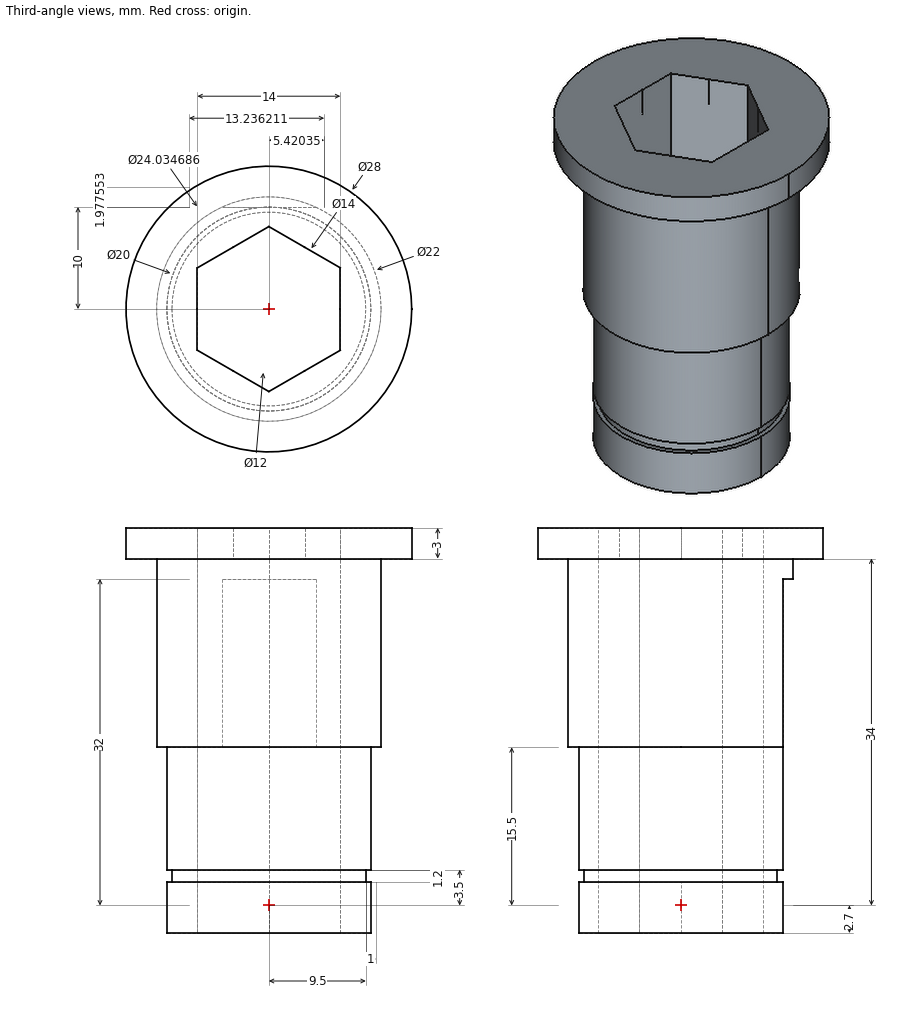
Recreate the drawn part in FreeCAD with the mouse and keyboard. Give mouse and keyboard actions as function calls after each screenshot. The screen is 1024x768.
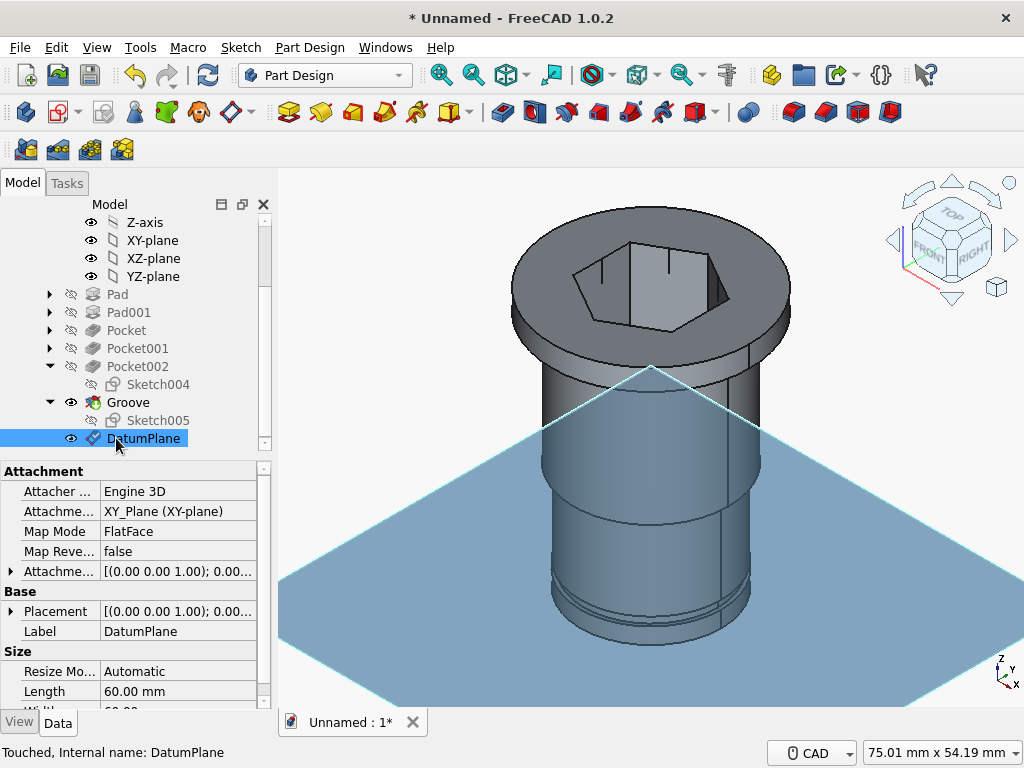
click(58, 112)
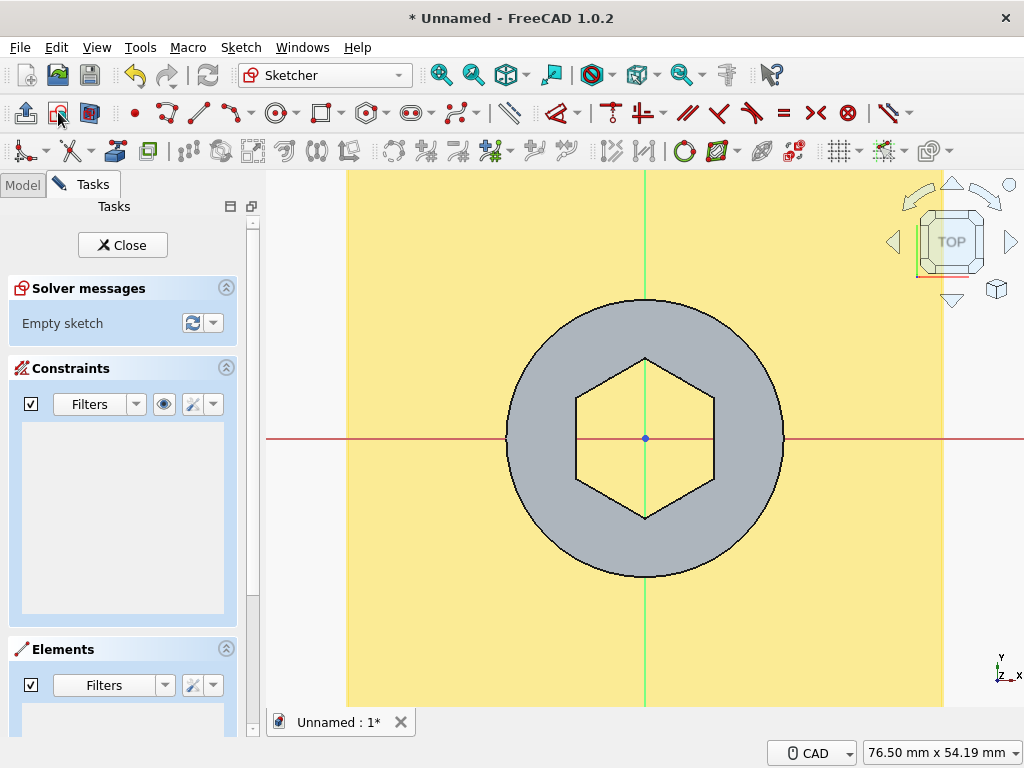
click(90, 114)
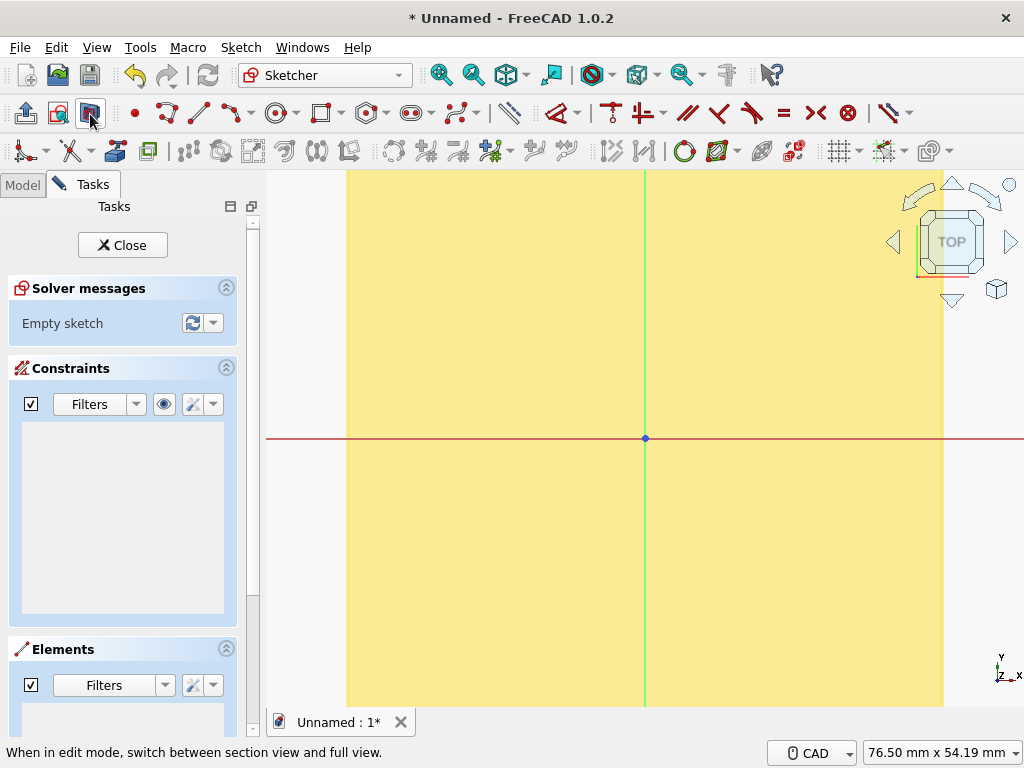
scroll(728, 438, up, 3)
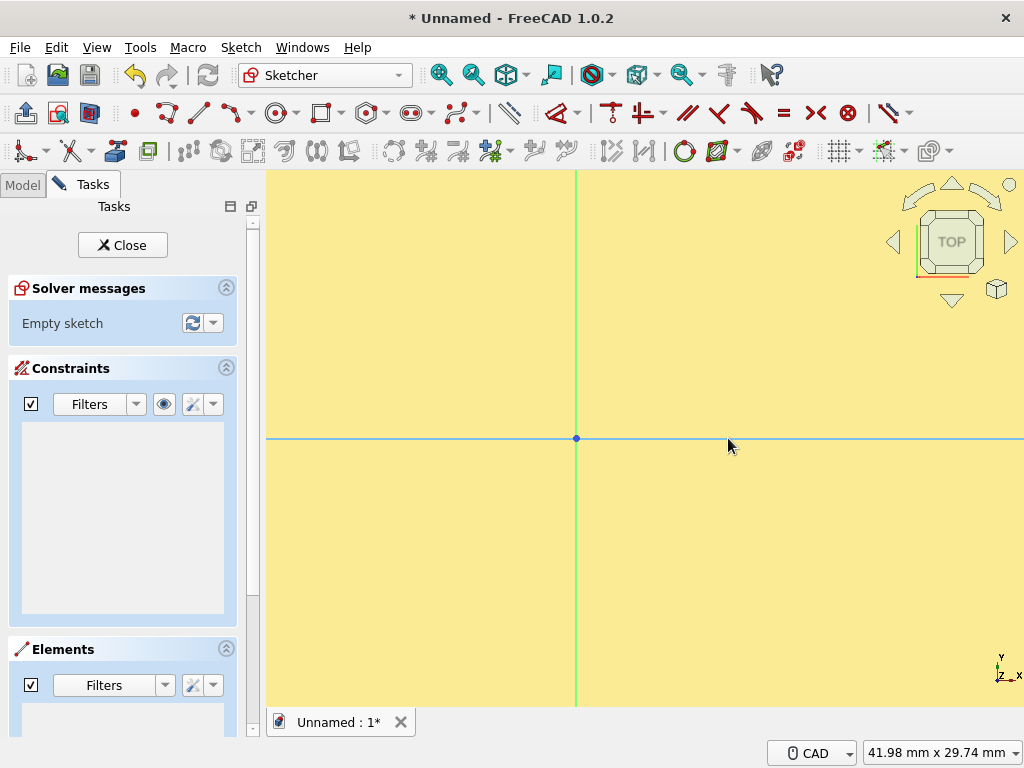
click(366, 114)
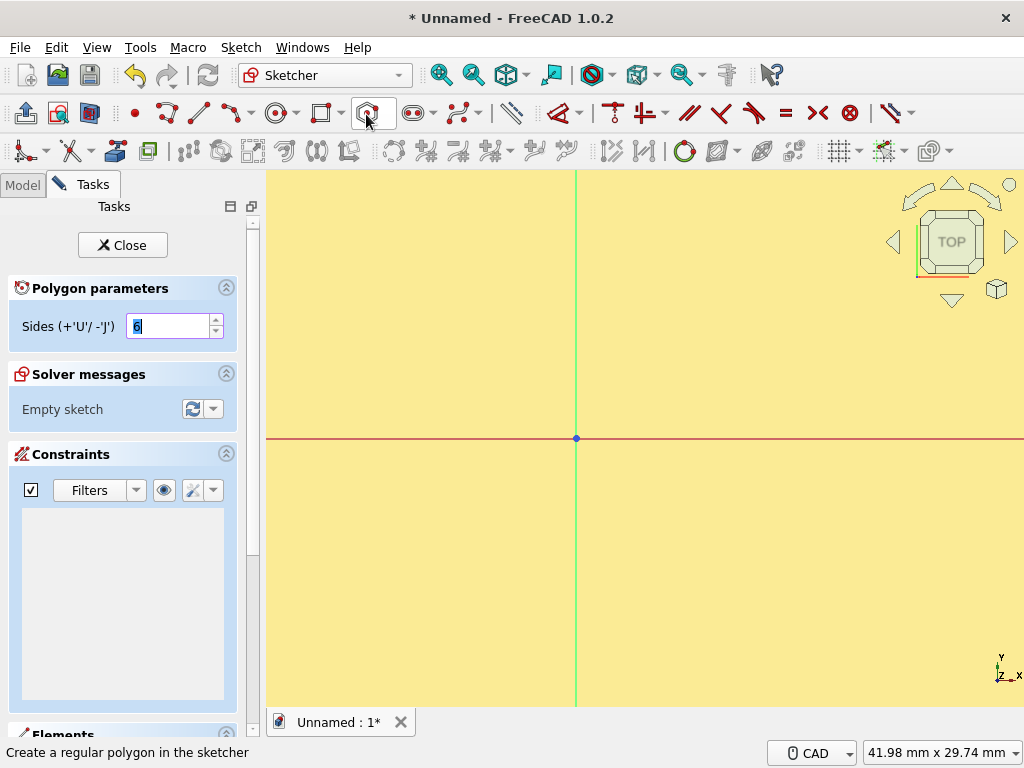
click(576, 438)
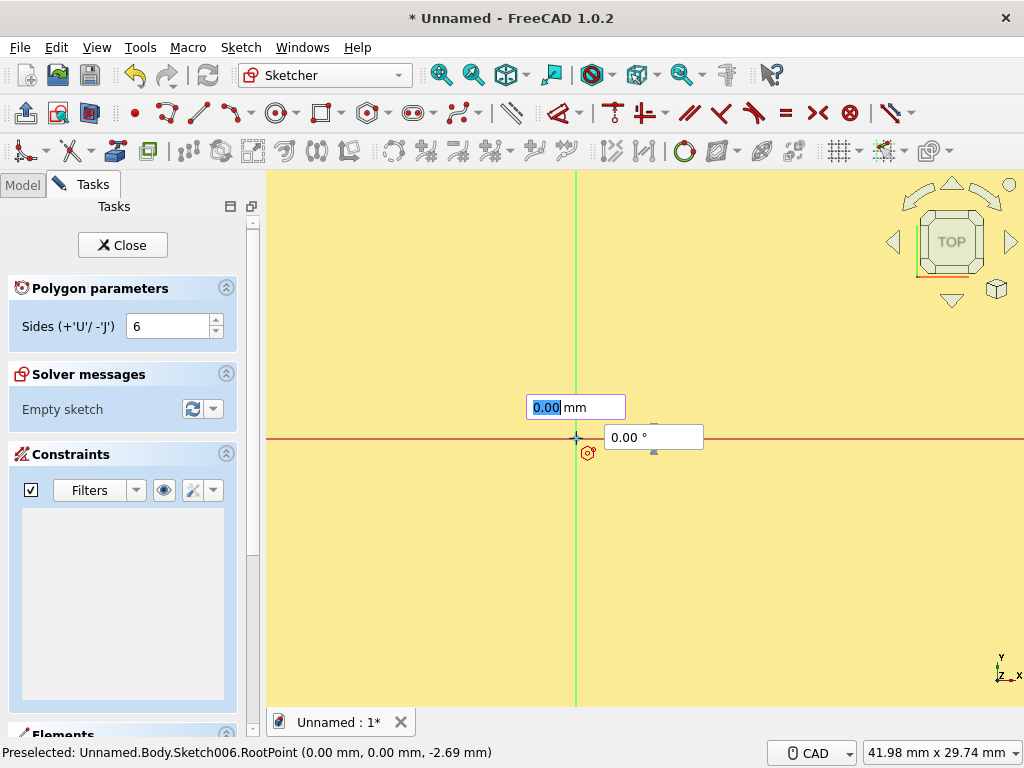
click(576, 584)
right_click(576, 584)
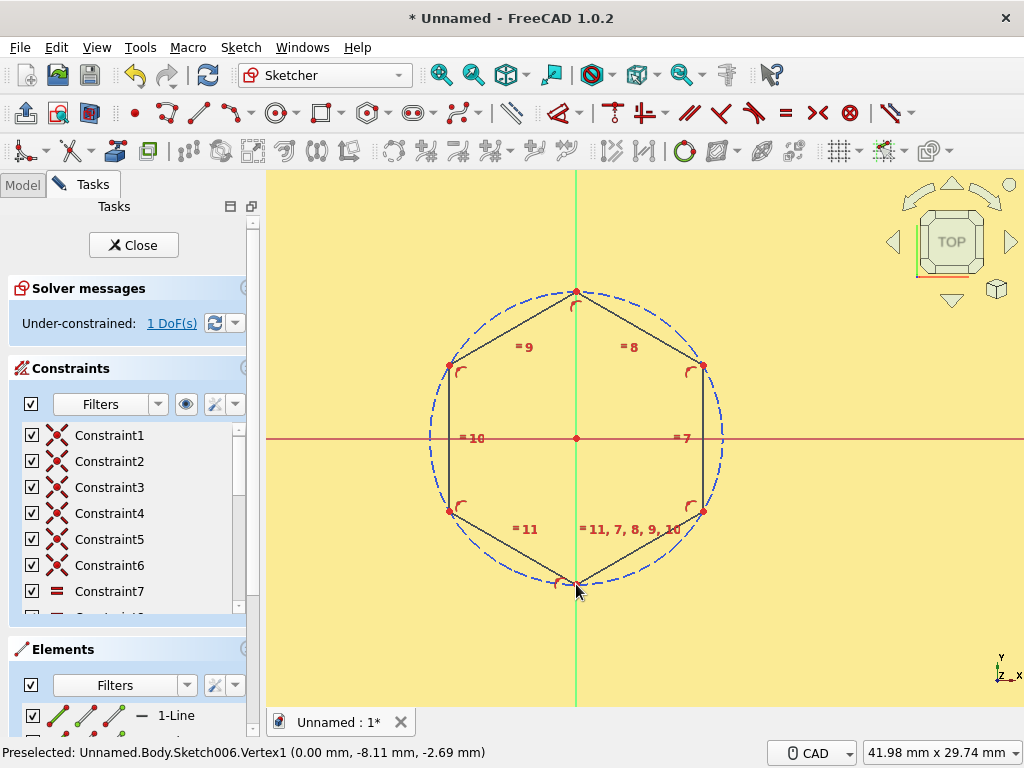
click(276, 114)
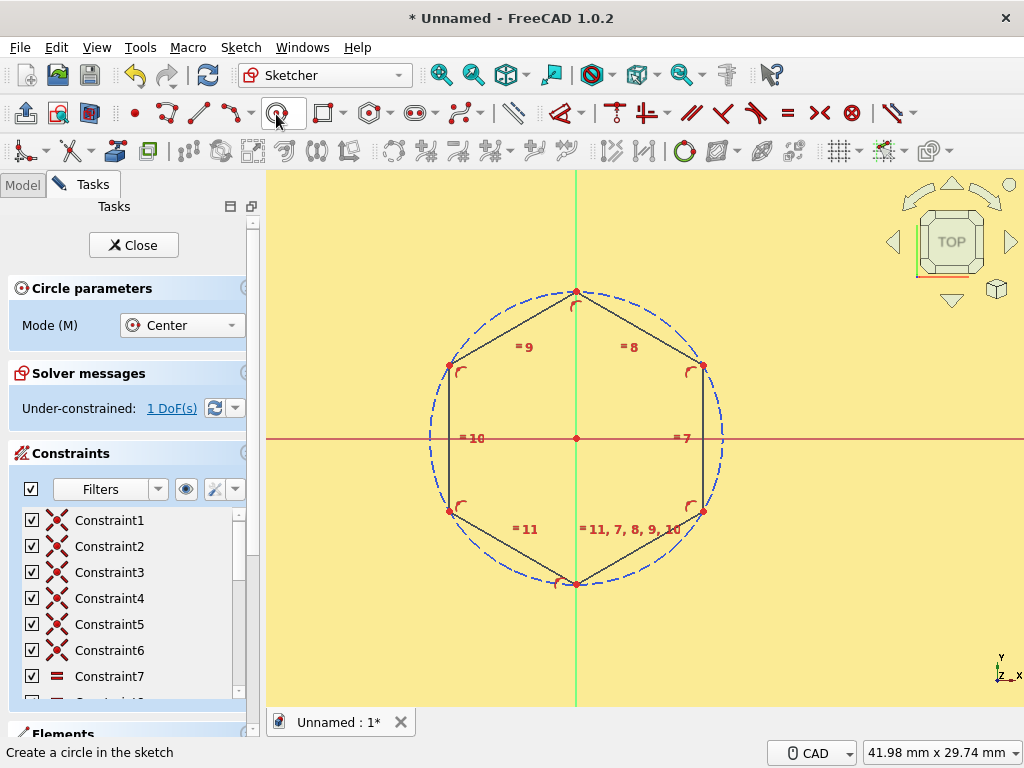
click(576, 438)
click(704, 311)
key(Escape)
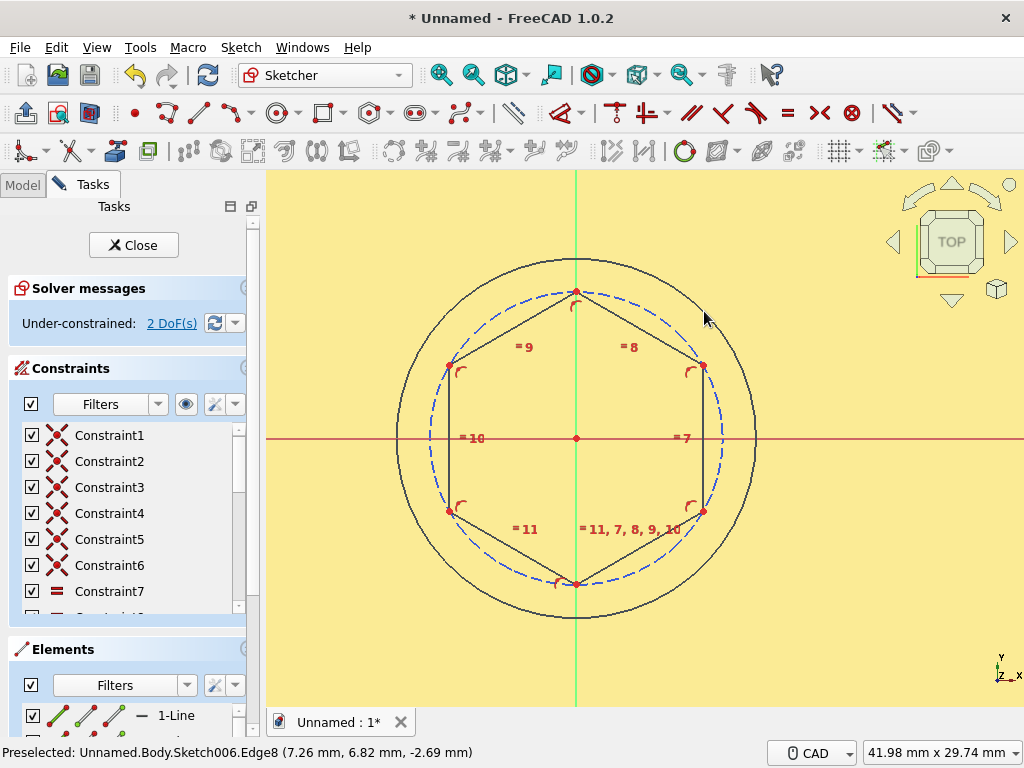
click(560, 114)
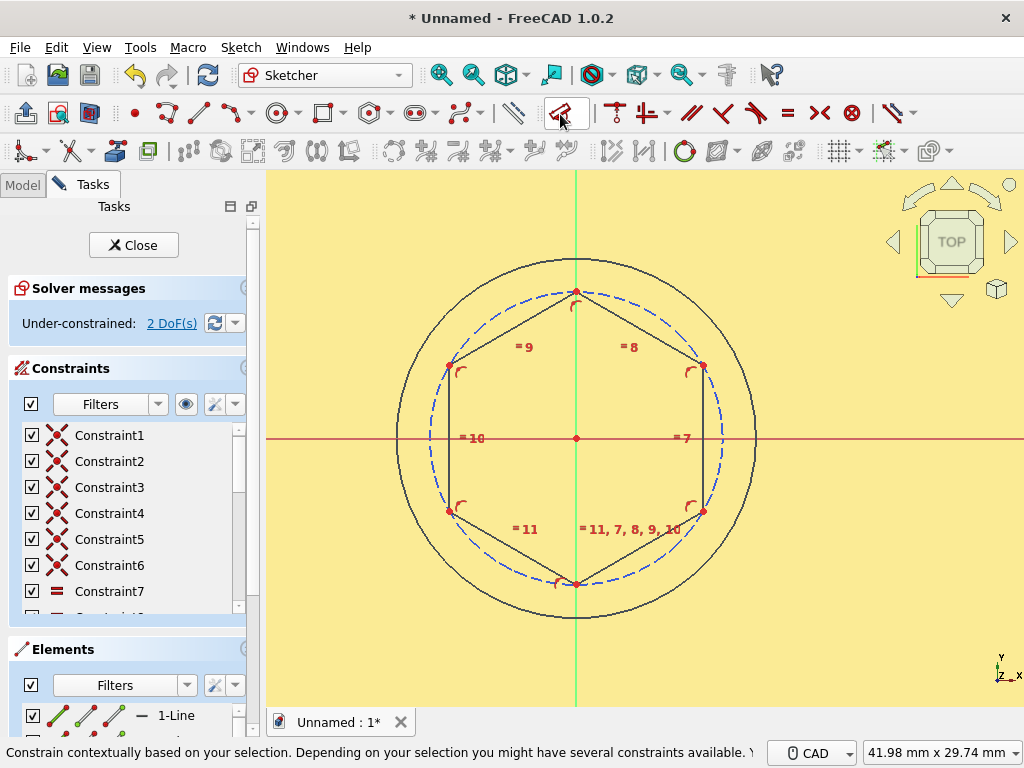
click(703, 311)
click(726, 288)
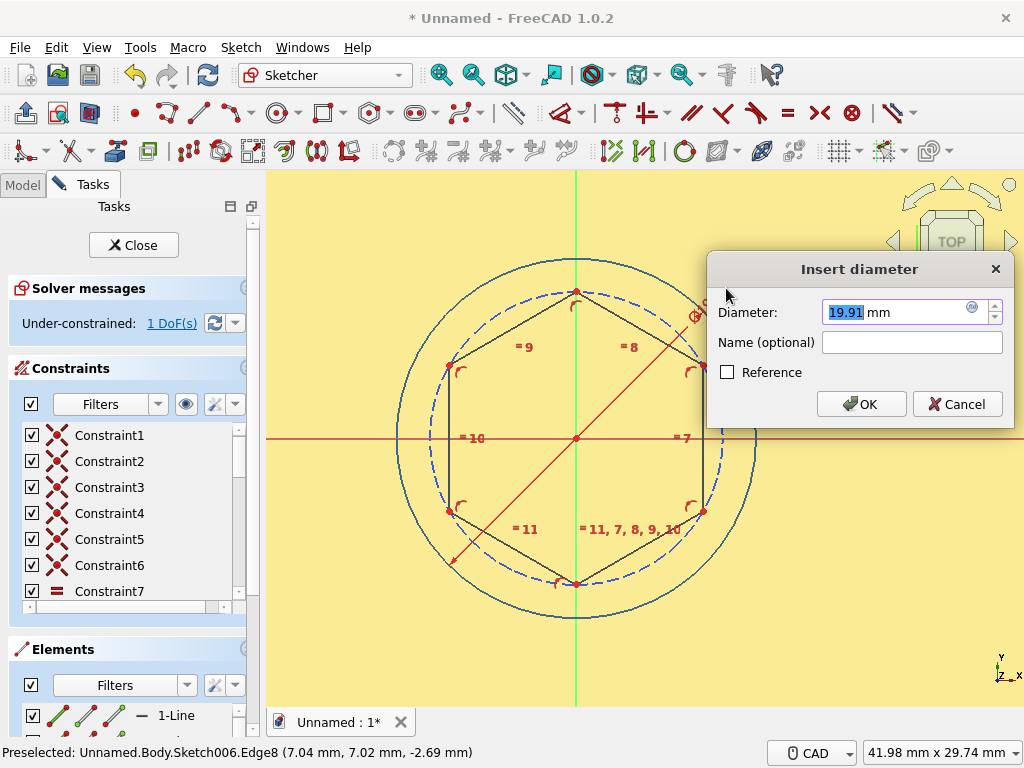
text(20)
key(Return)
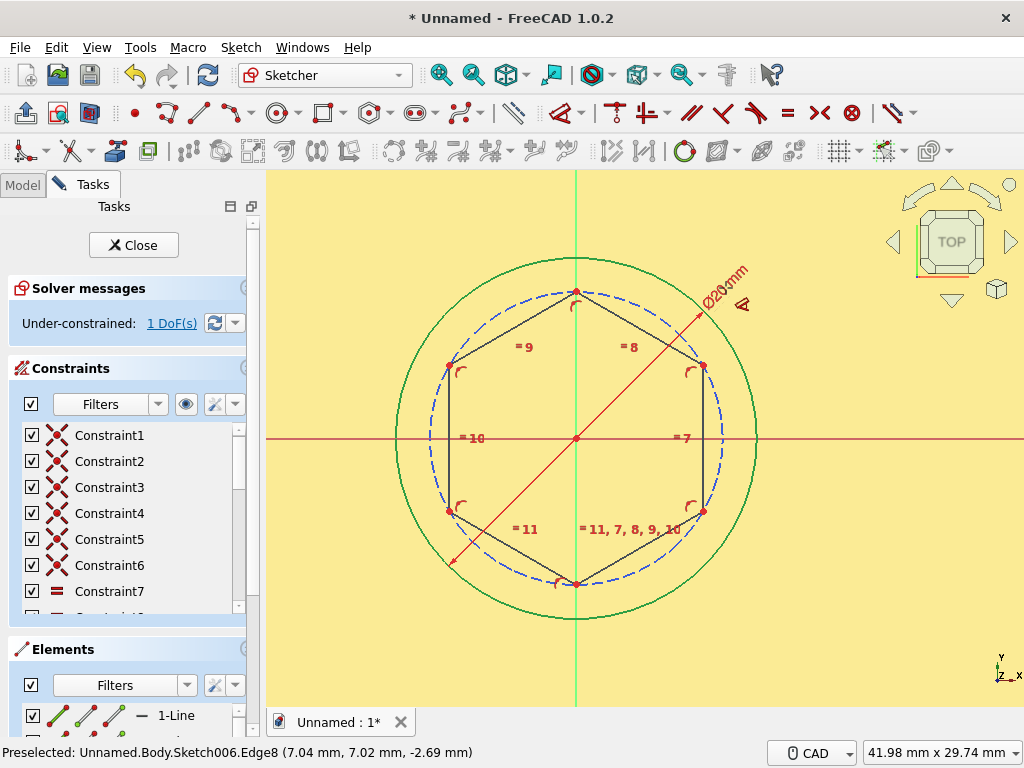
click(449, 365)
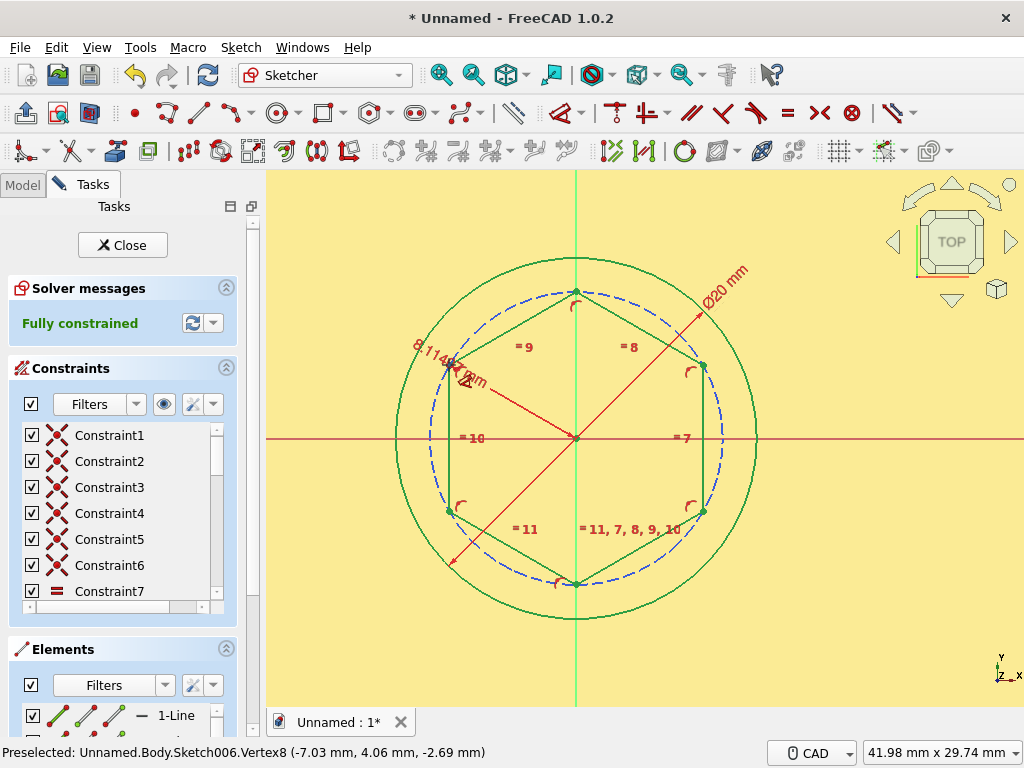
click(703, 512)
click(518, 594)